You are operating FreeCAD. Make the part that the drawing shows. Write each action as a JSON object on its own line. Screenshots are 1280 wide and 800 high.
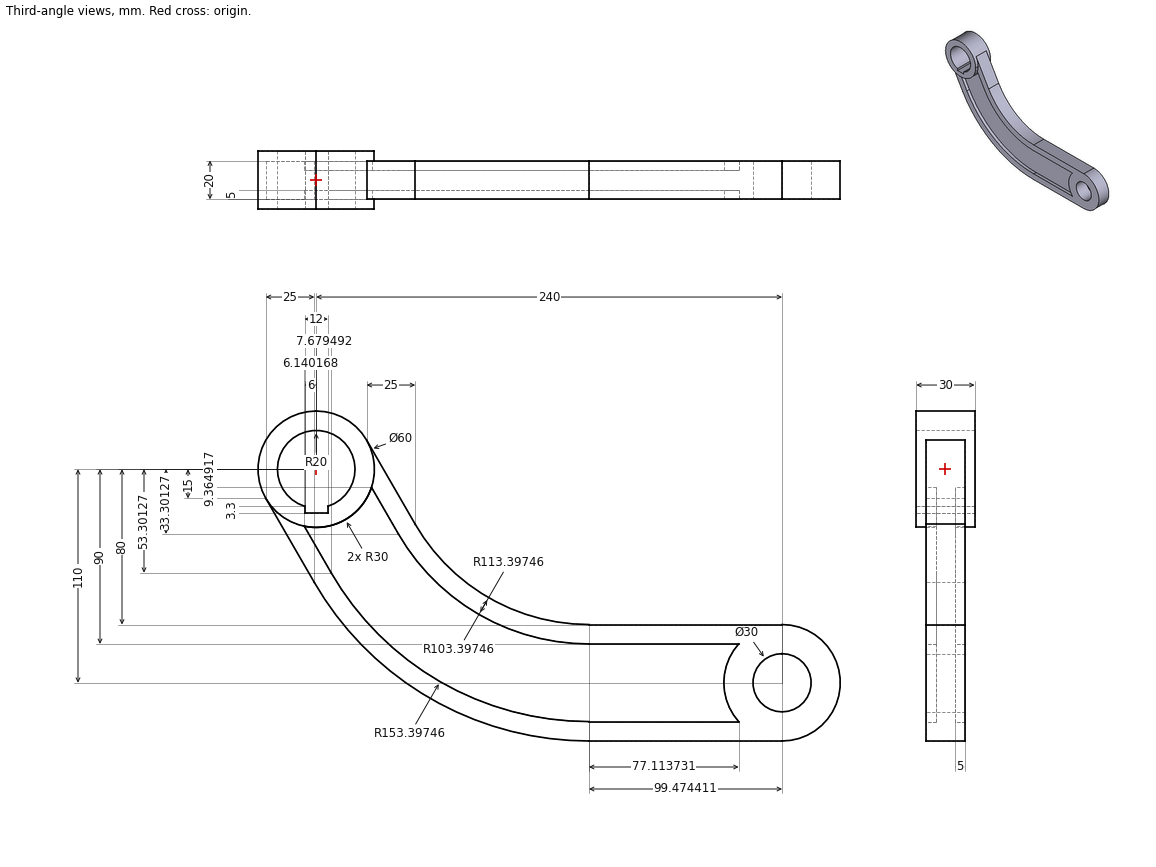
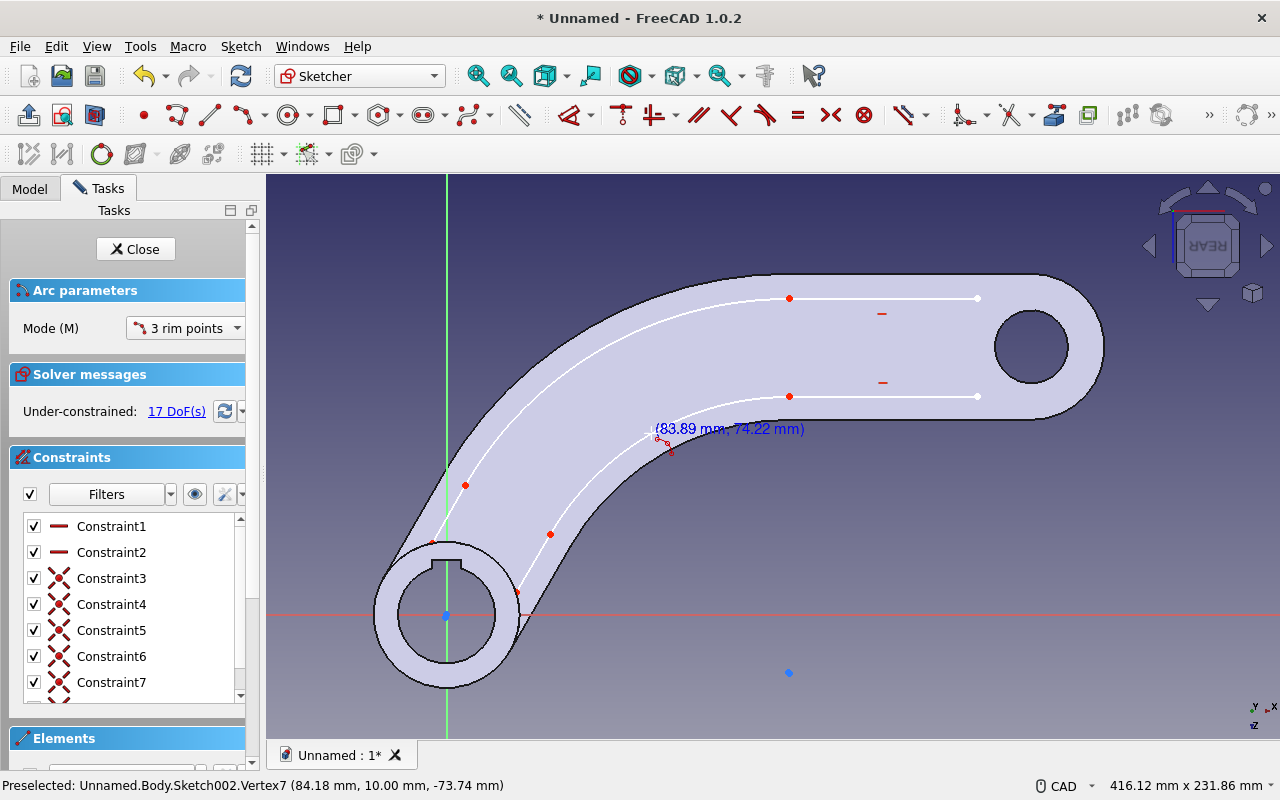
{"action": "left_click", "coordinate": [977, 397]}
{"action": "left_click", "coordinate": [977, 299]}
{"action": "left_click", "coordinate": [958, 347]}
{"action": "key", "text": "Escape"}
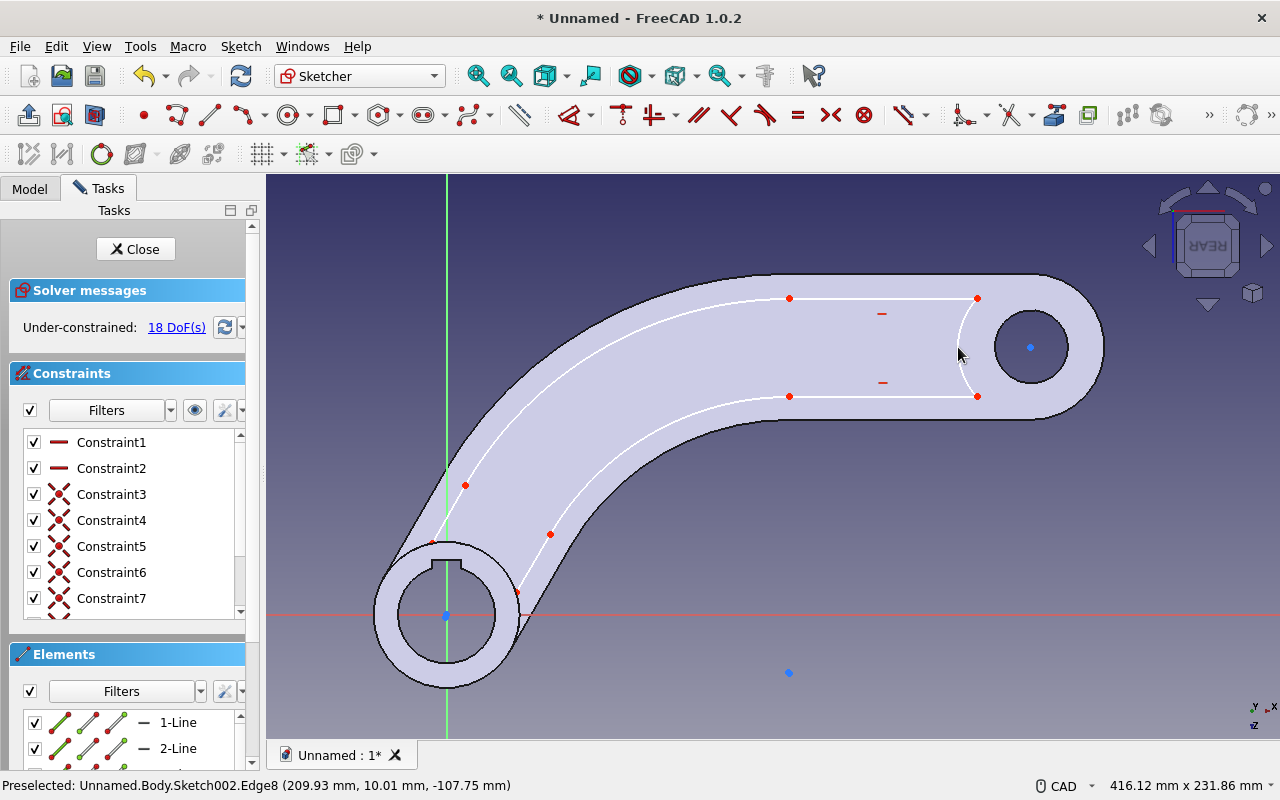
{"action": "left_click", "coordinate": [445, 521]}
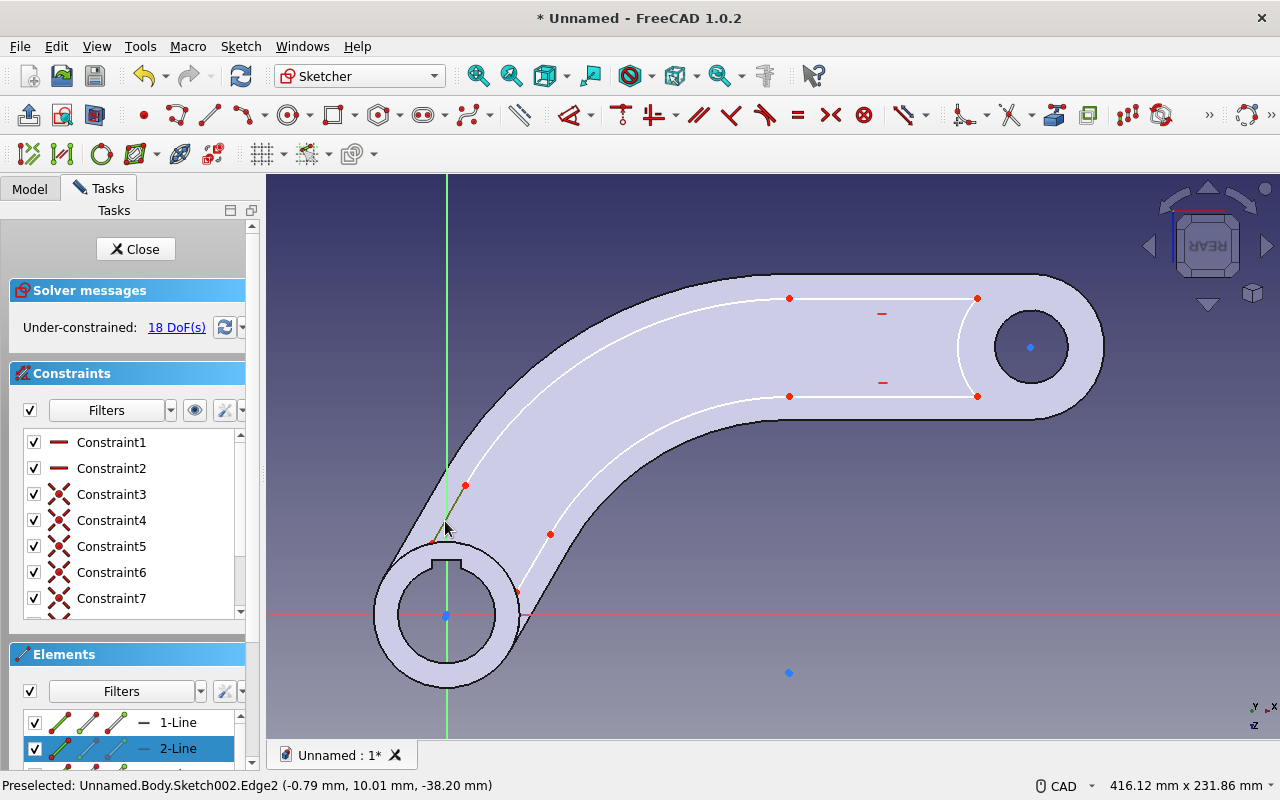
{"action": "left_click", "coordinate": [673, 317]}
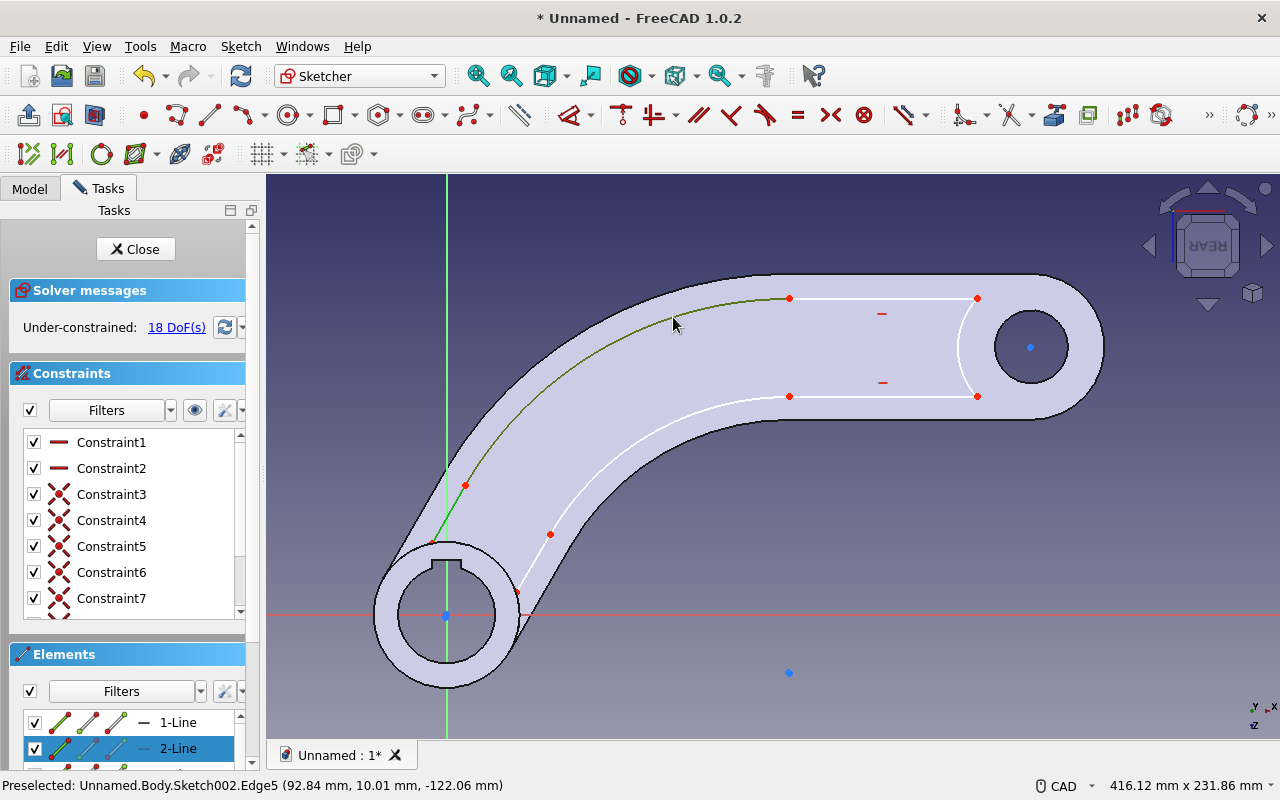
{"action": "left_click", "coordinate": [765, 116]}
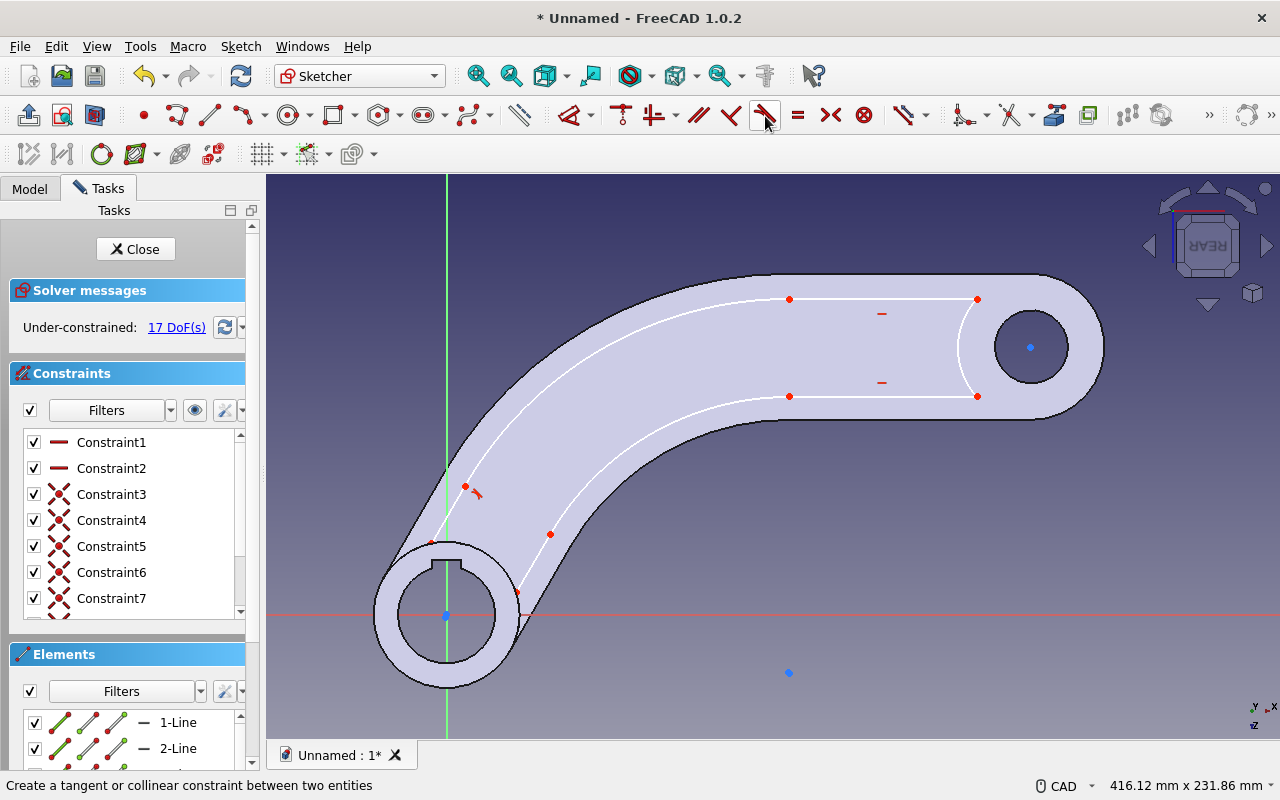
{"action": "left_click", "coordinate": [526, 576]}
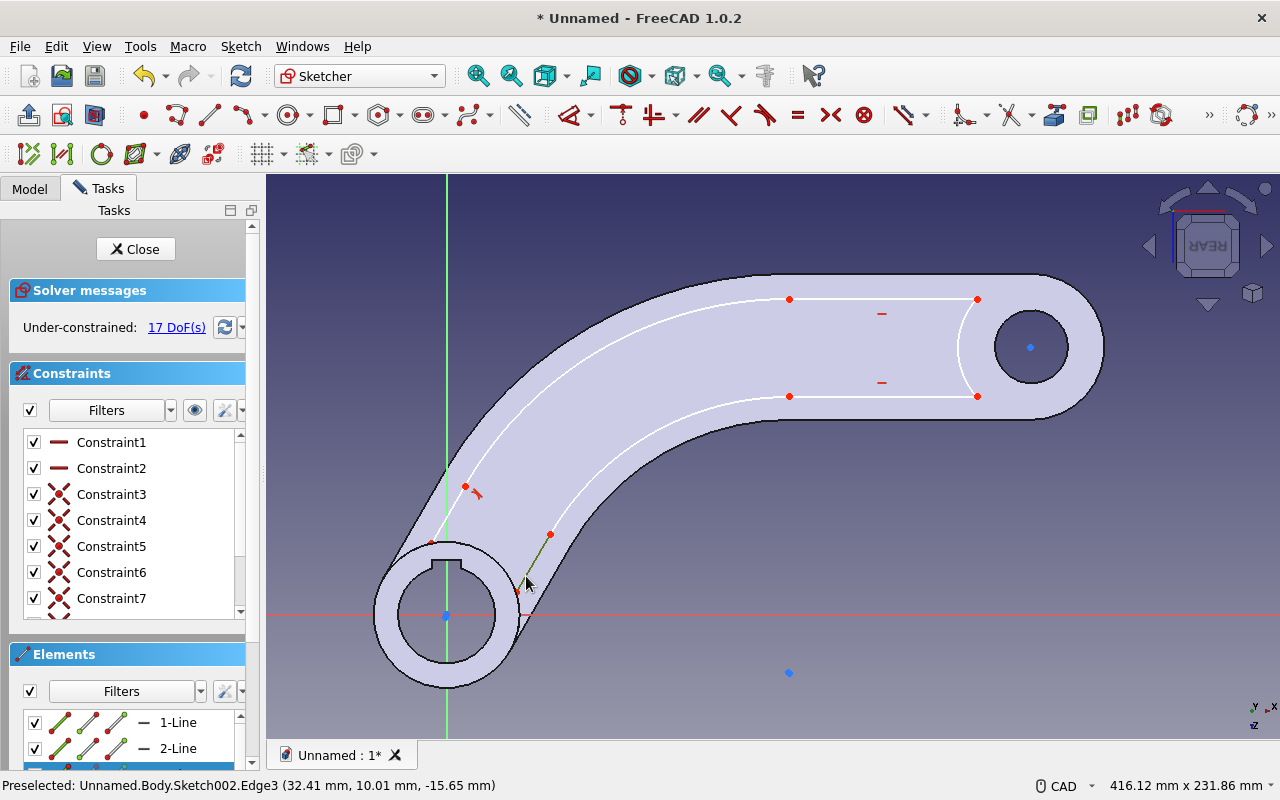
{"action": "left_click", "coordinate": [704, 411]}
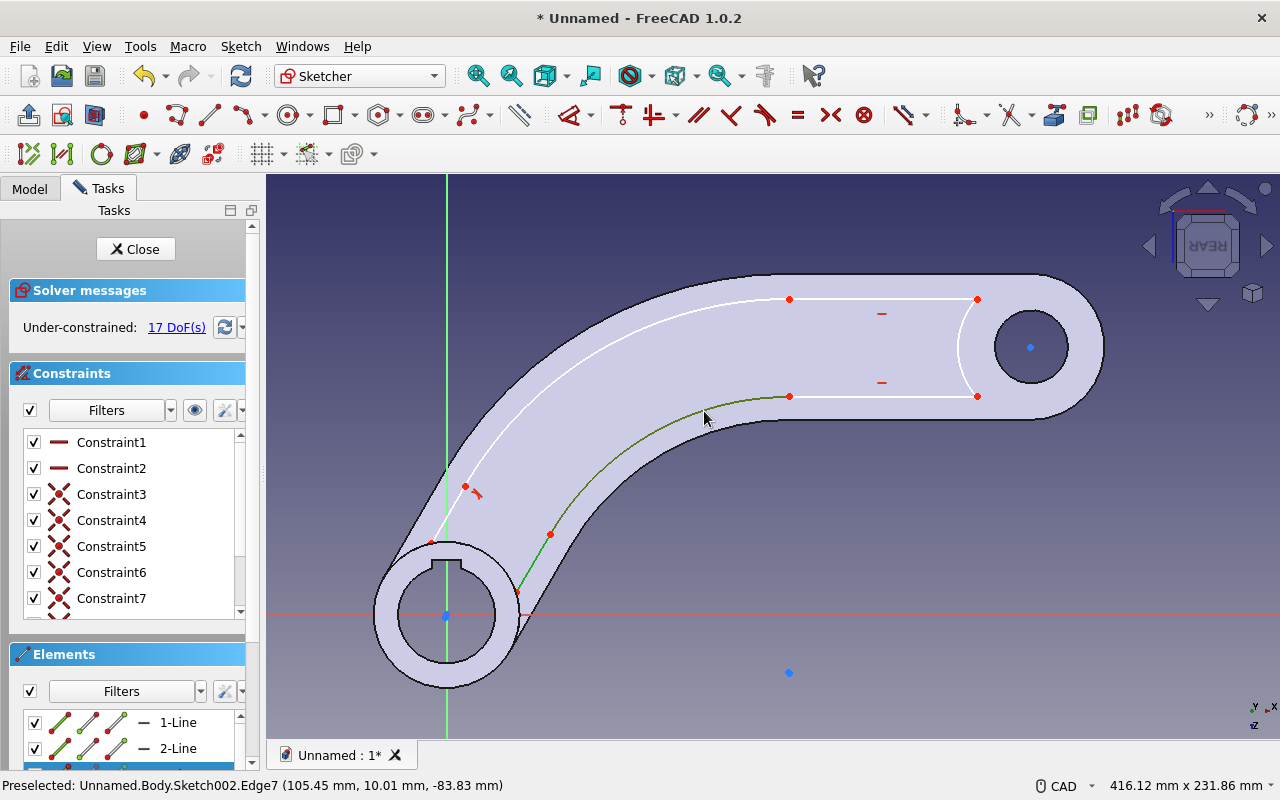
{"action": "left_click", "coordinate": [765, 116]}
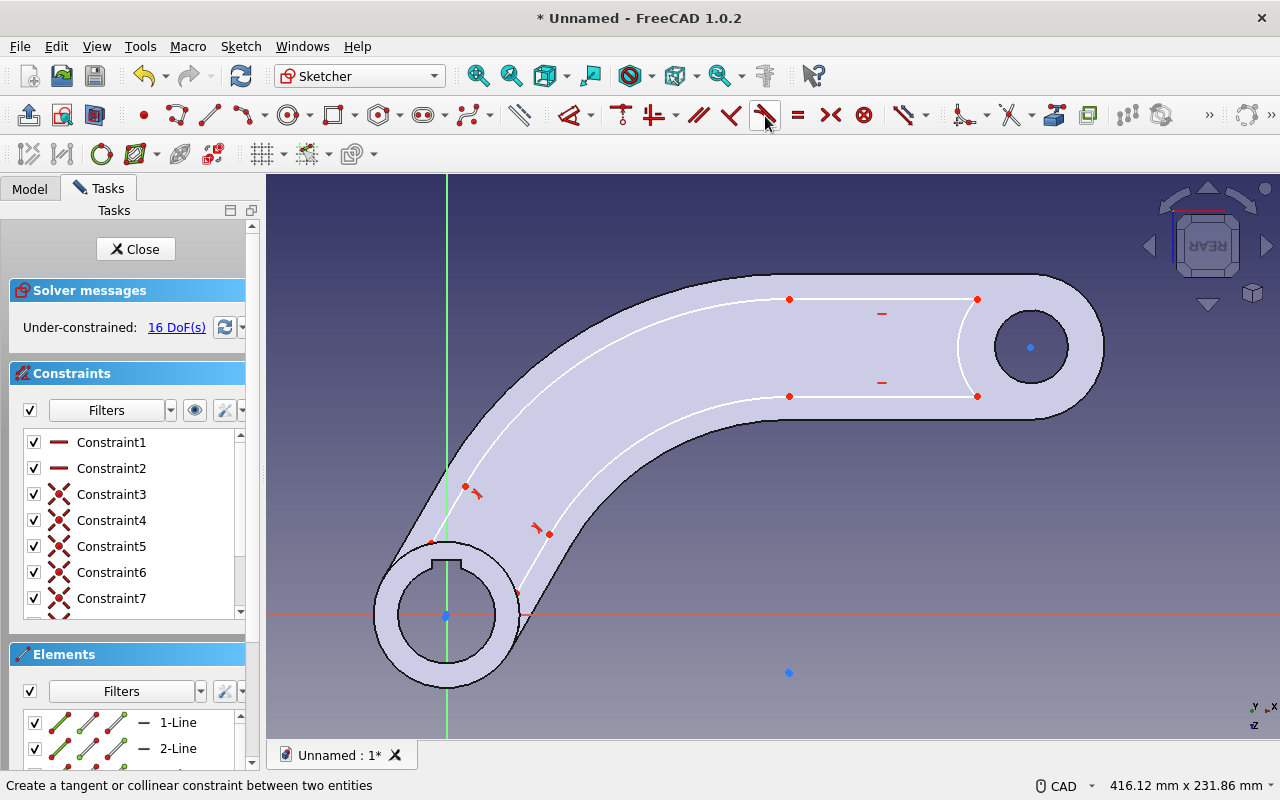
{"action": "left_click", "coordinate": [673, 317]}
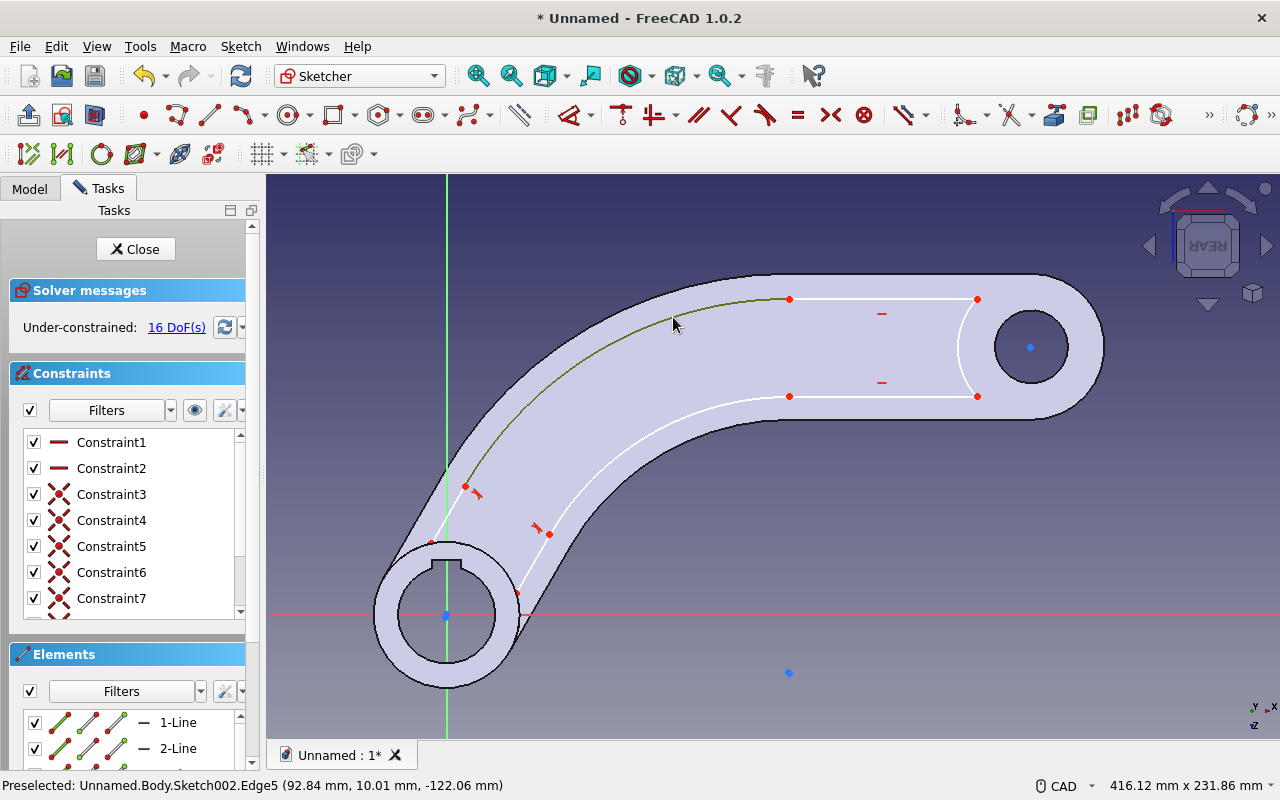
{"action": "left_click", "coordinate": [704, 411]}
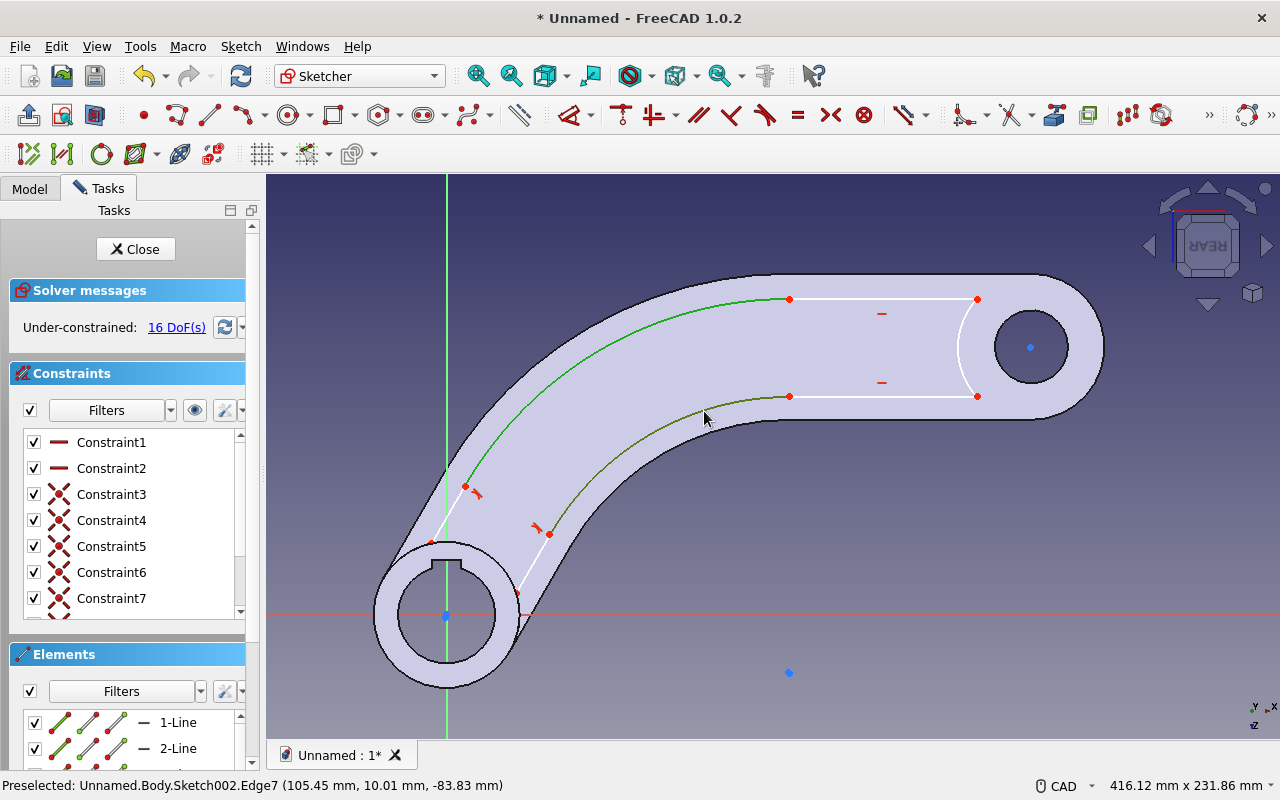
{"action": "left_click", "coordinate": [621, 116]}